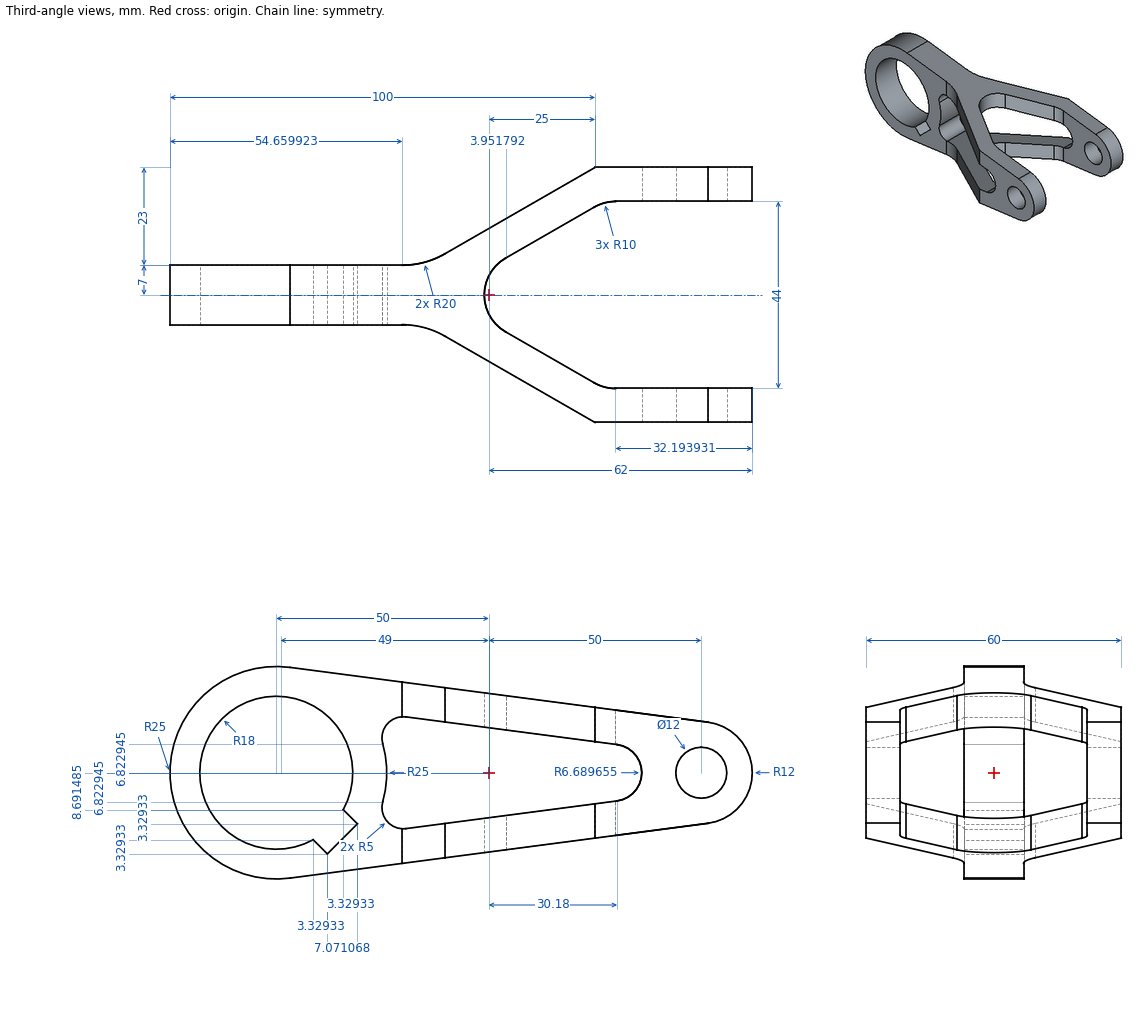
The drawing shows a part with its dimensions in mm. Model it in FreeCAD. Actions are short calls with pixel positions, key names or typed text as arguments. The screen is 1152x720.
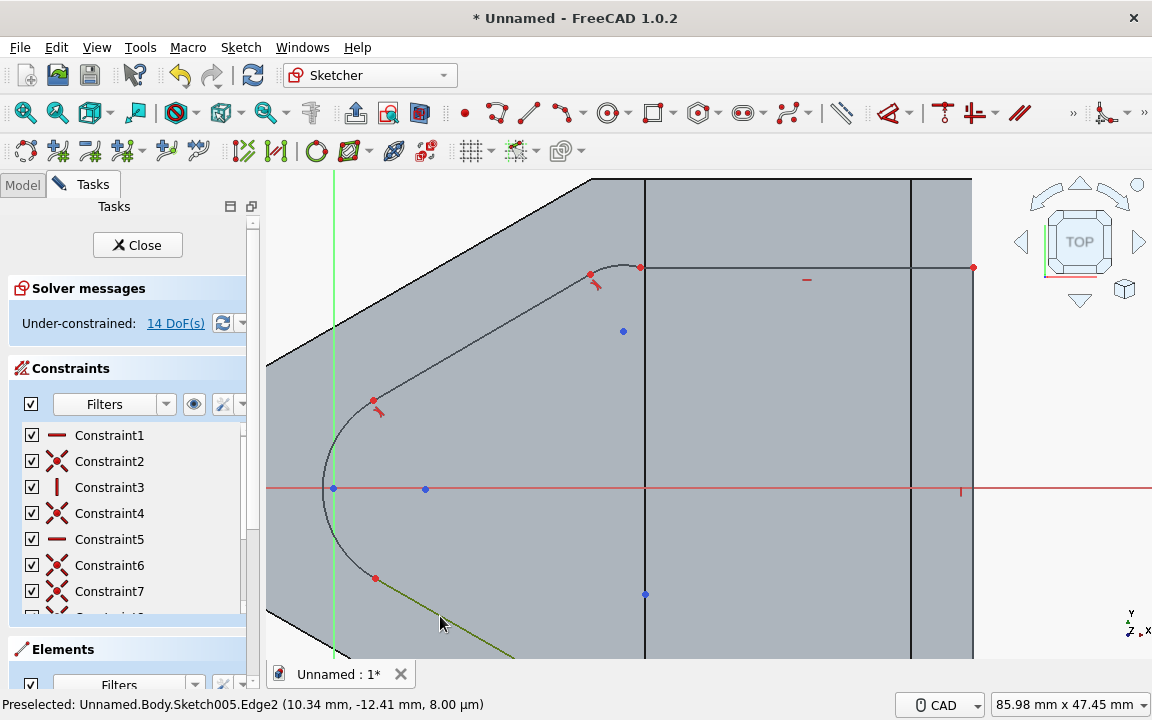
click(331, 448)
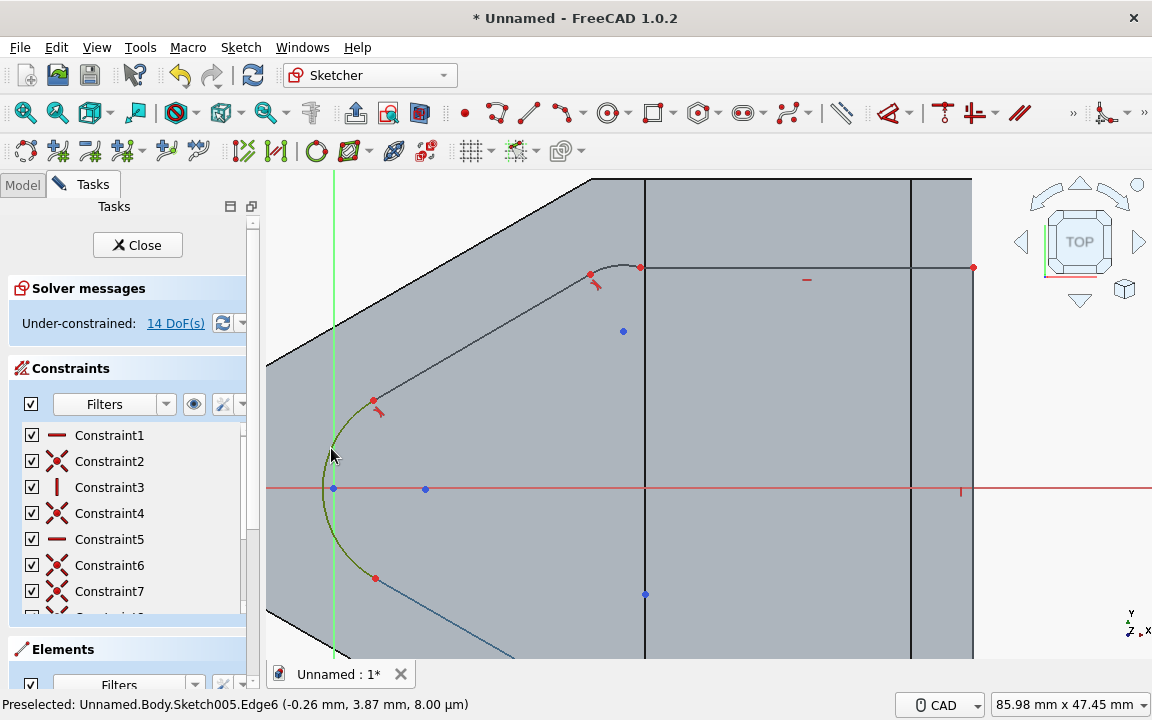
key(t)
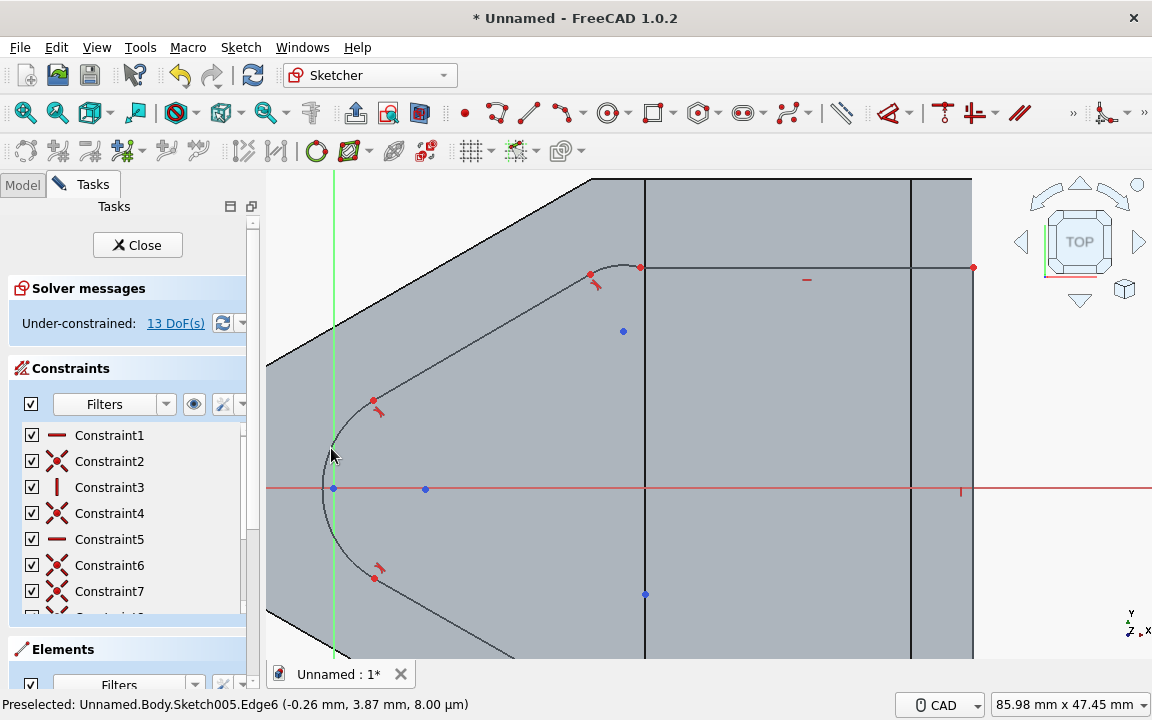
click(439, 616)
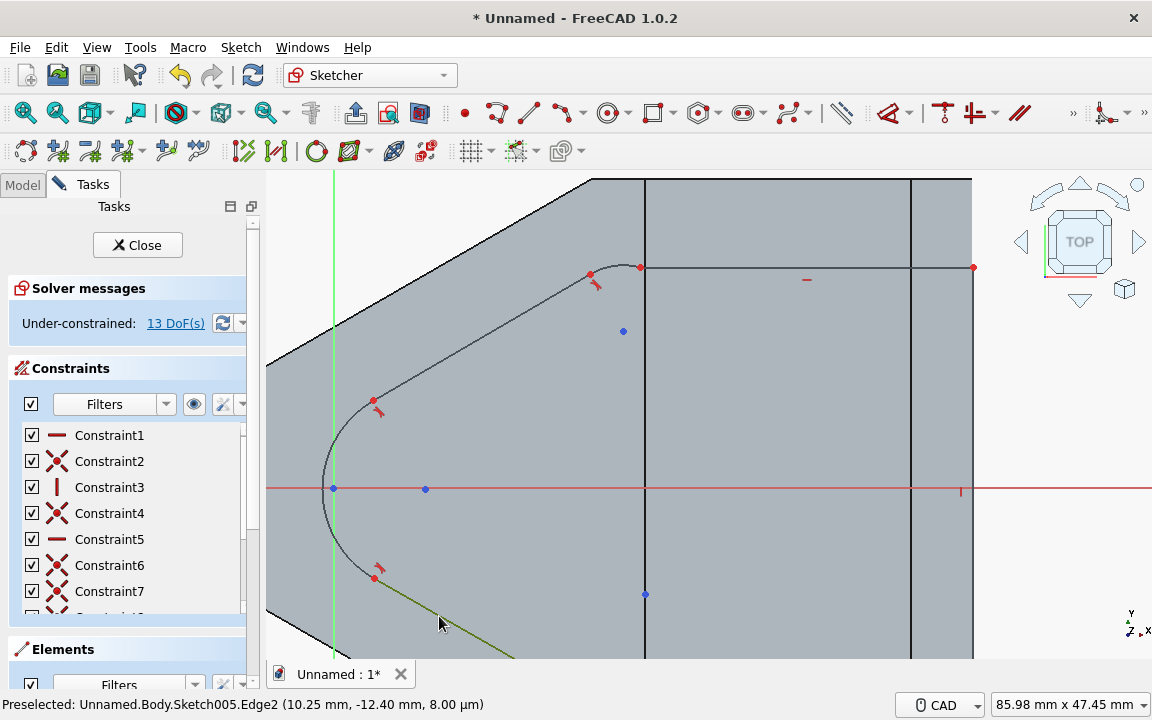
scroll(625, 265, down, 2)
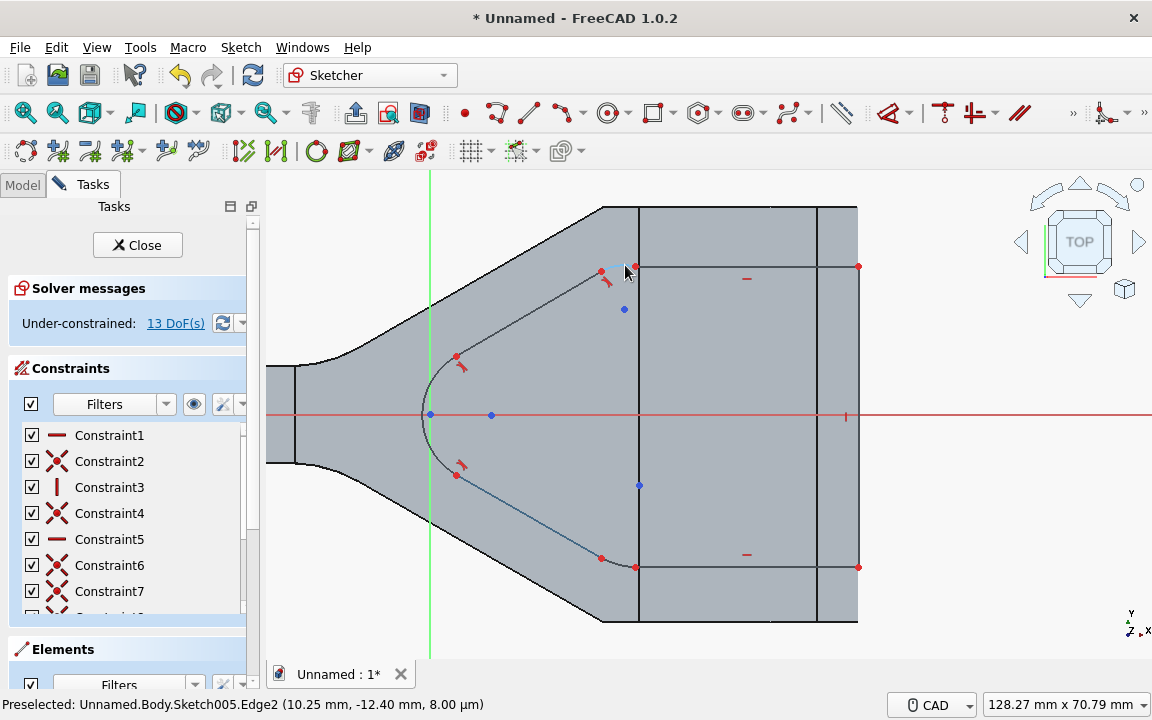
scroll(611, 562, up, 2)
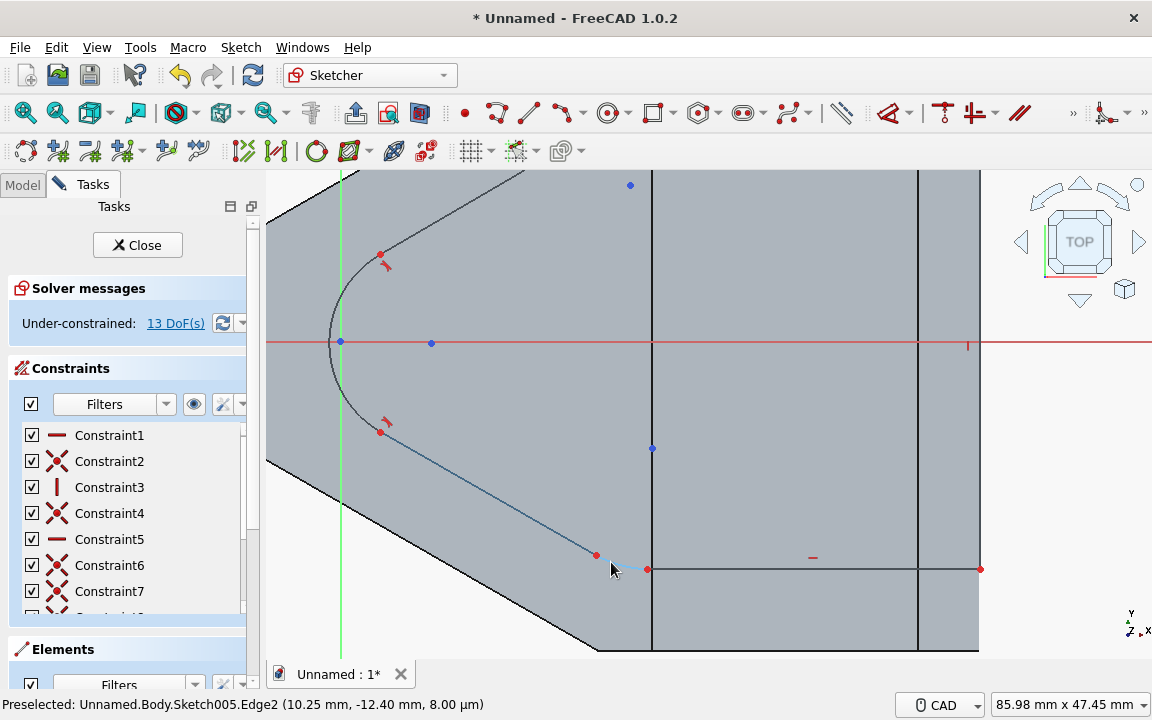
click(611, 562)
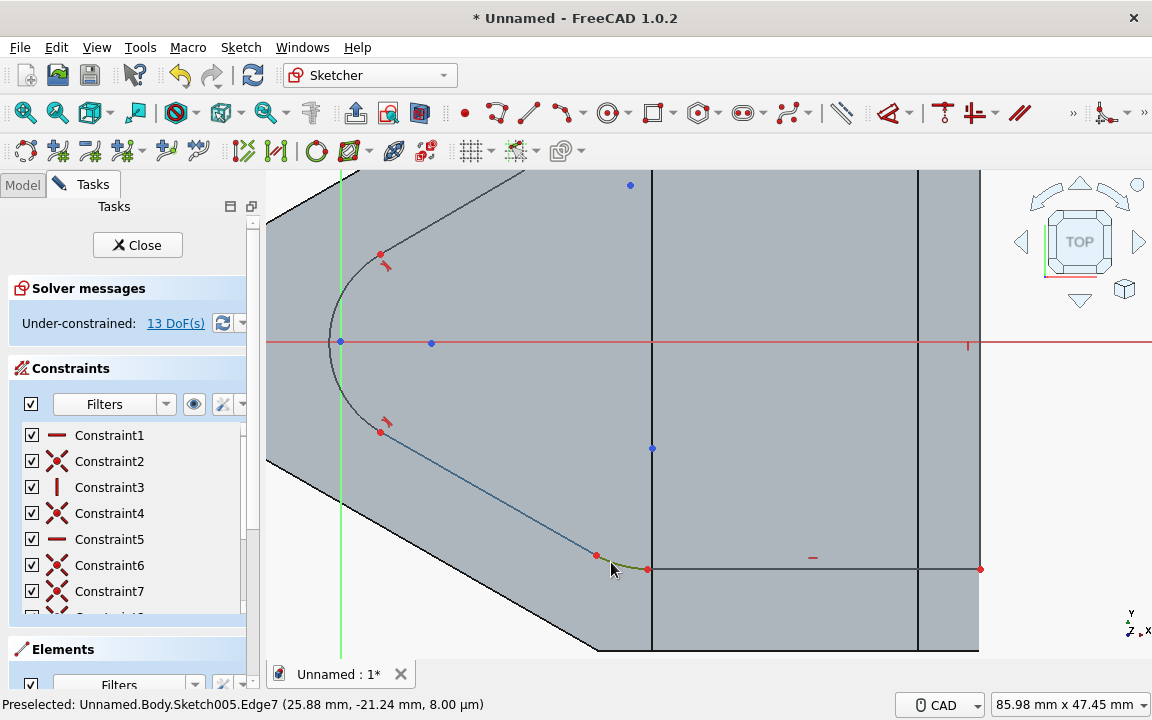
key(t)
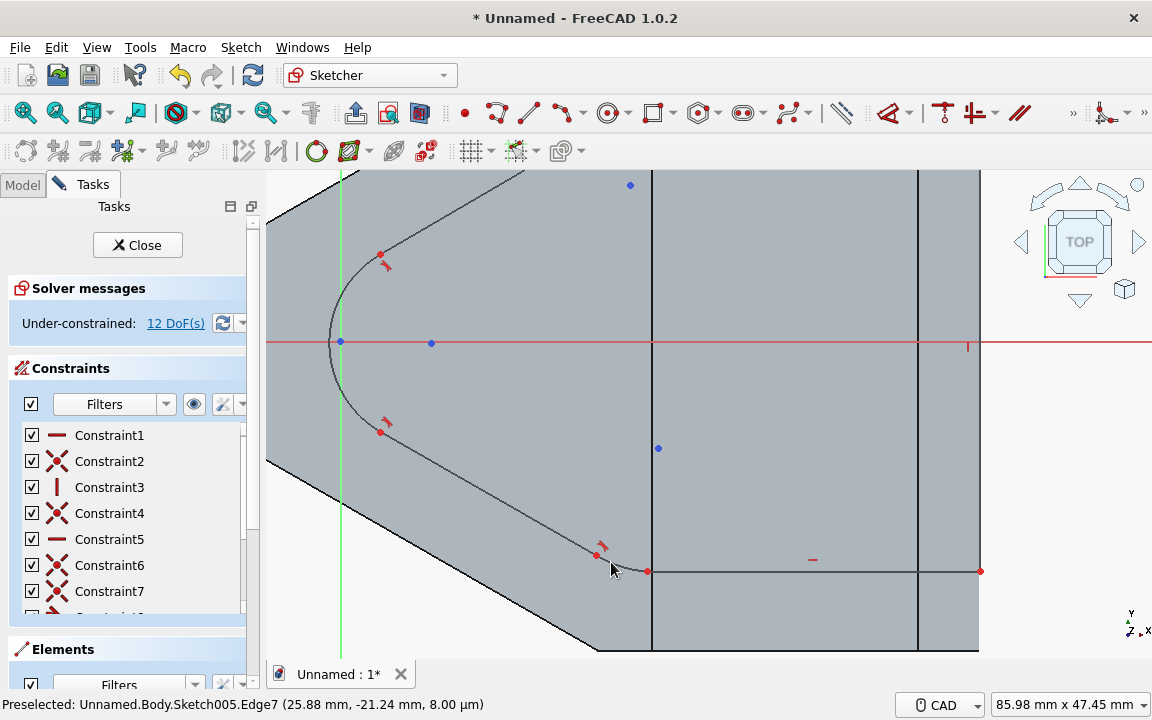
click(747, 572)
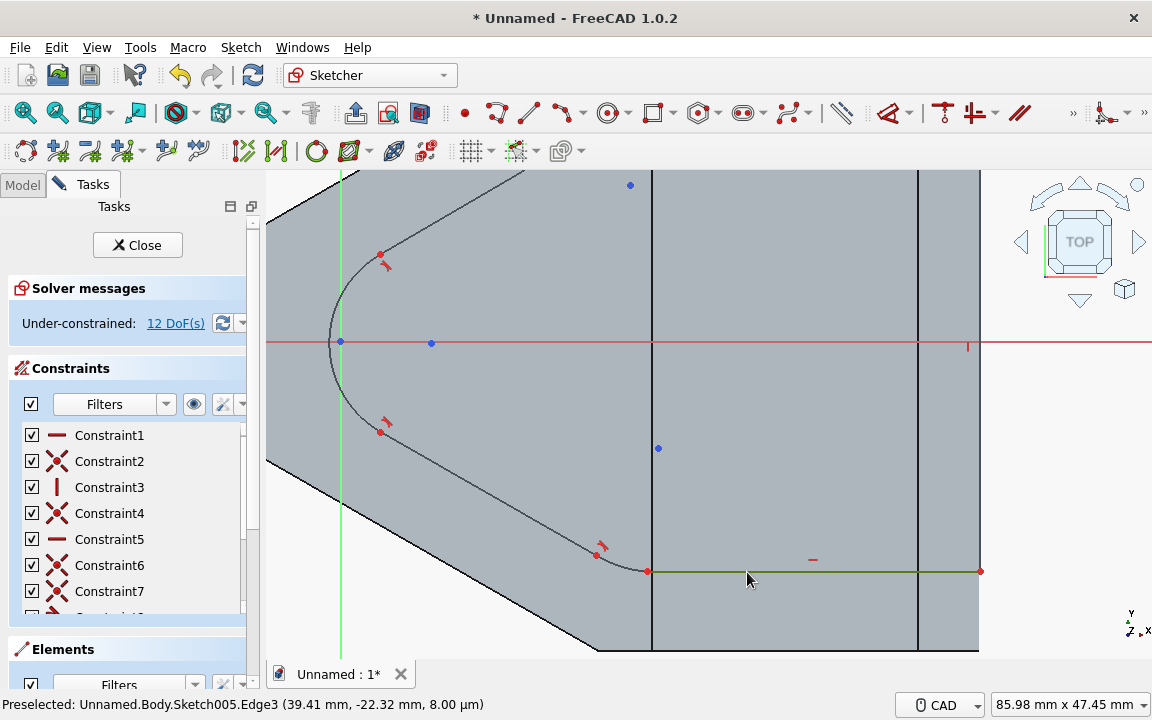
click(611, 563)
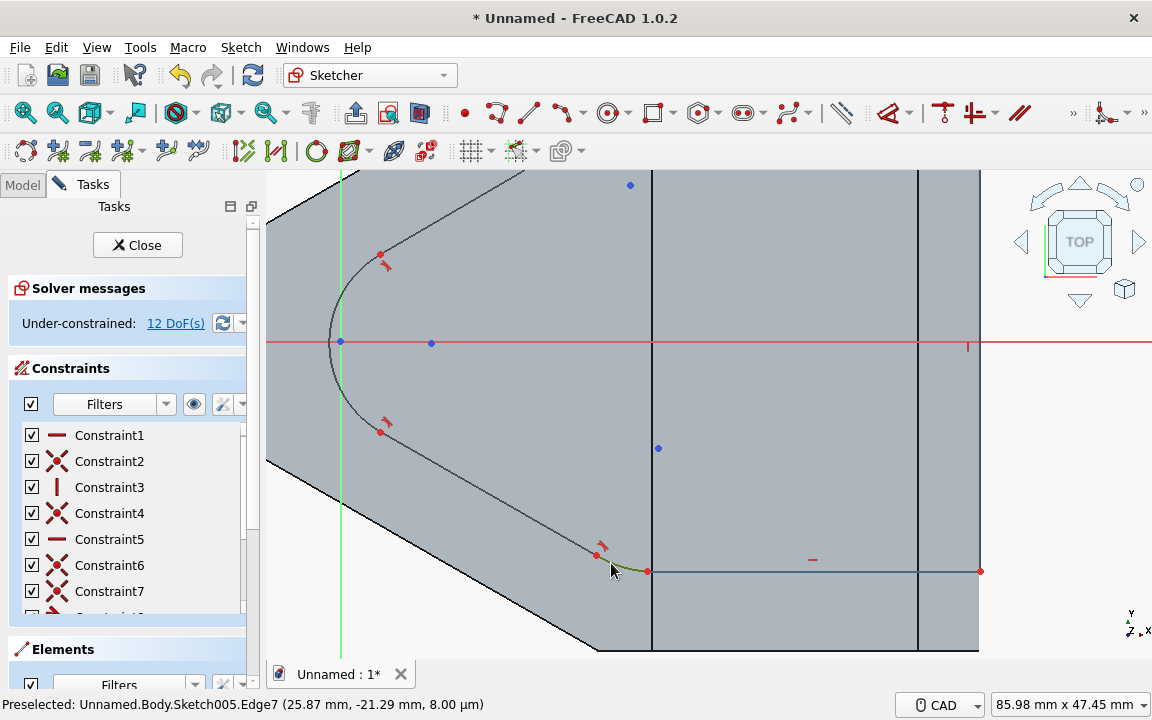
key(t)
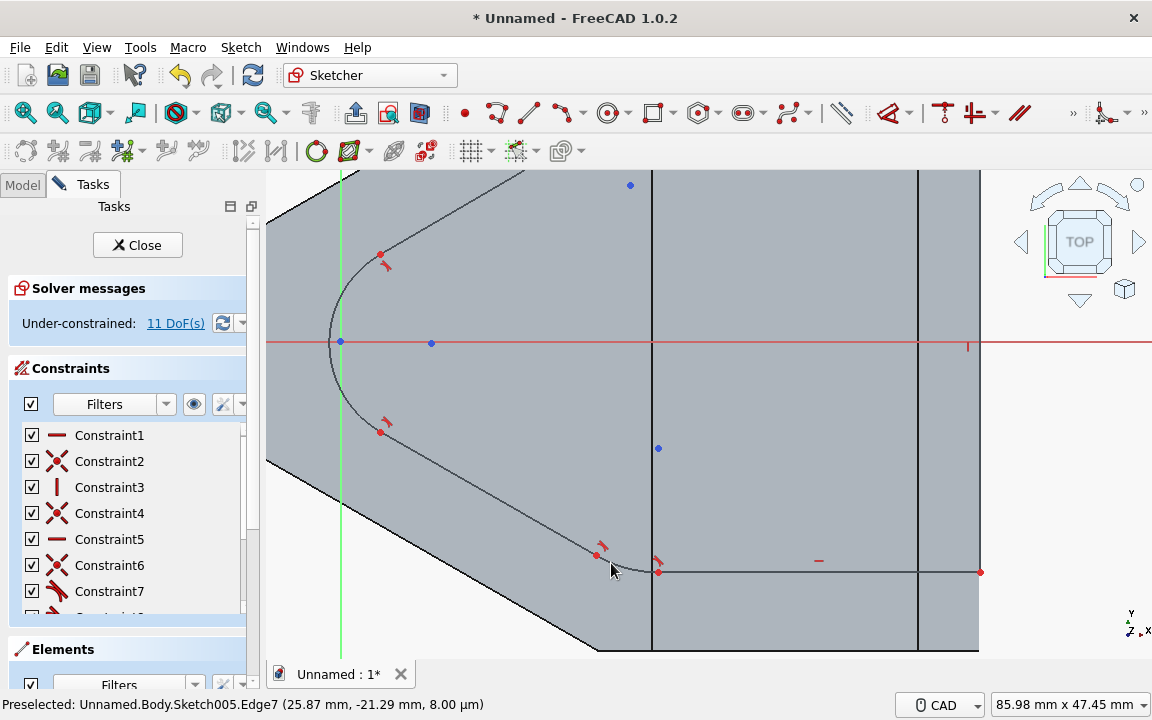
scroll(611, 562, down, 2)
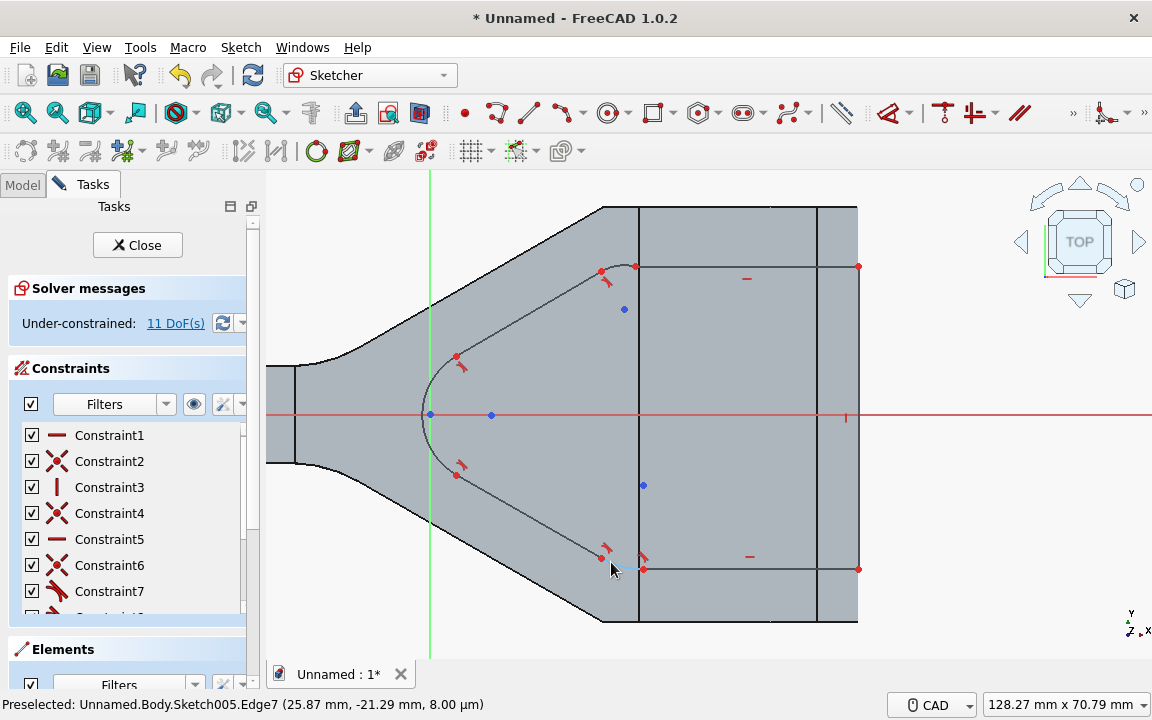
click(792, 267)